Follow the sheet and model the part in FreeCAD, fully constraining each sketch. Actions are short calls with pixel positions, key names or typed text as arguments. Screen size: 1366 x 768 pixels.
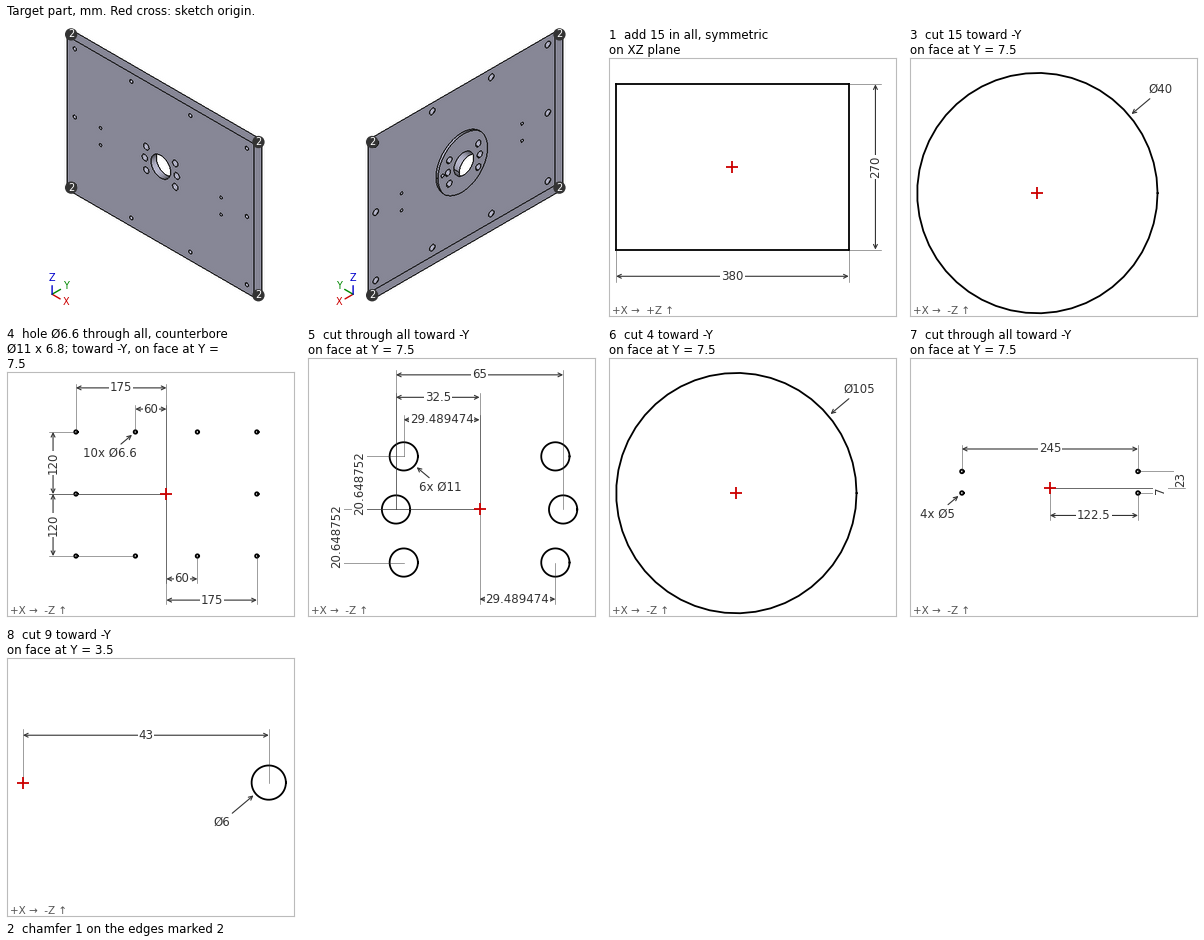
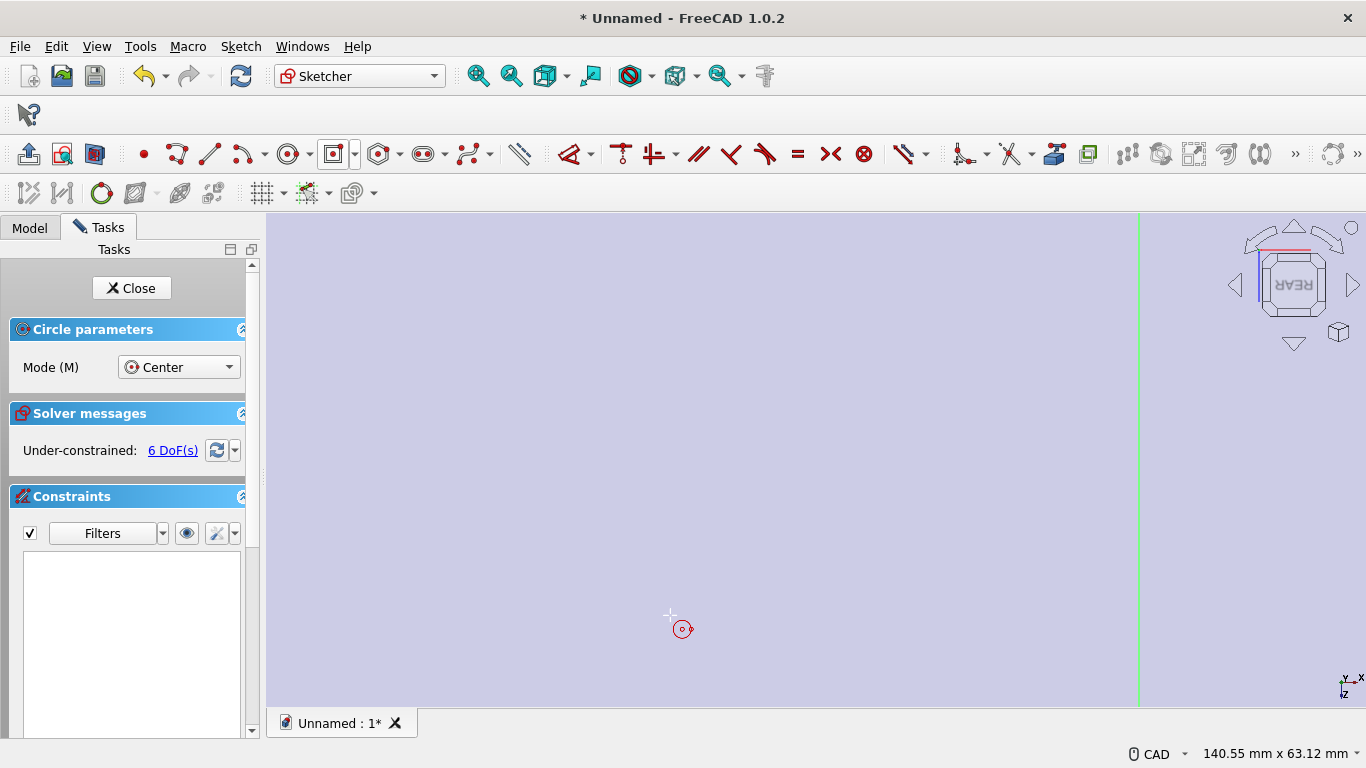
scroll(670, 616, down, 9)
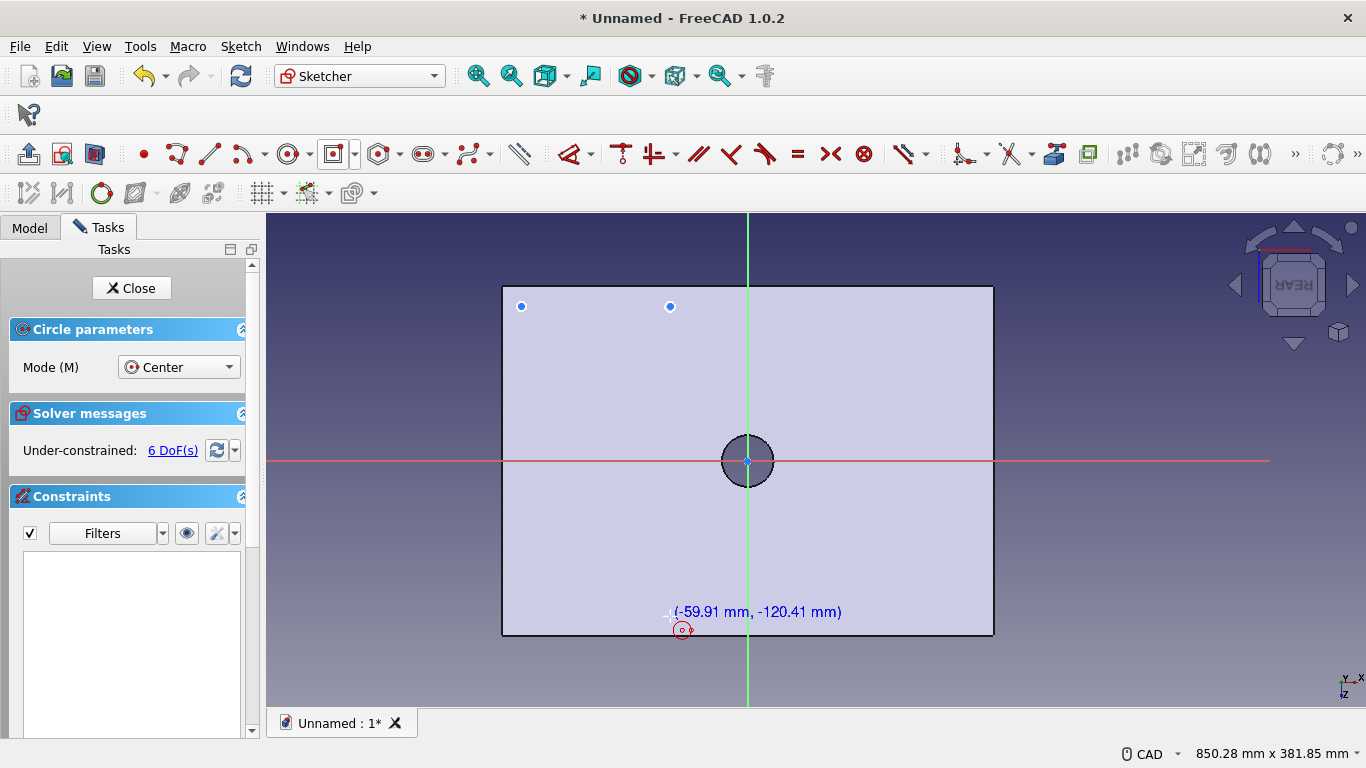
click(670, 616)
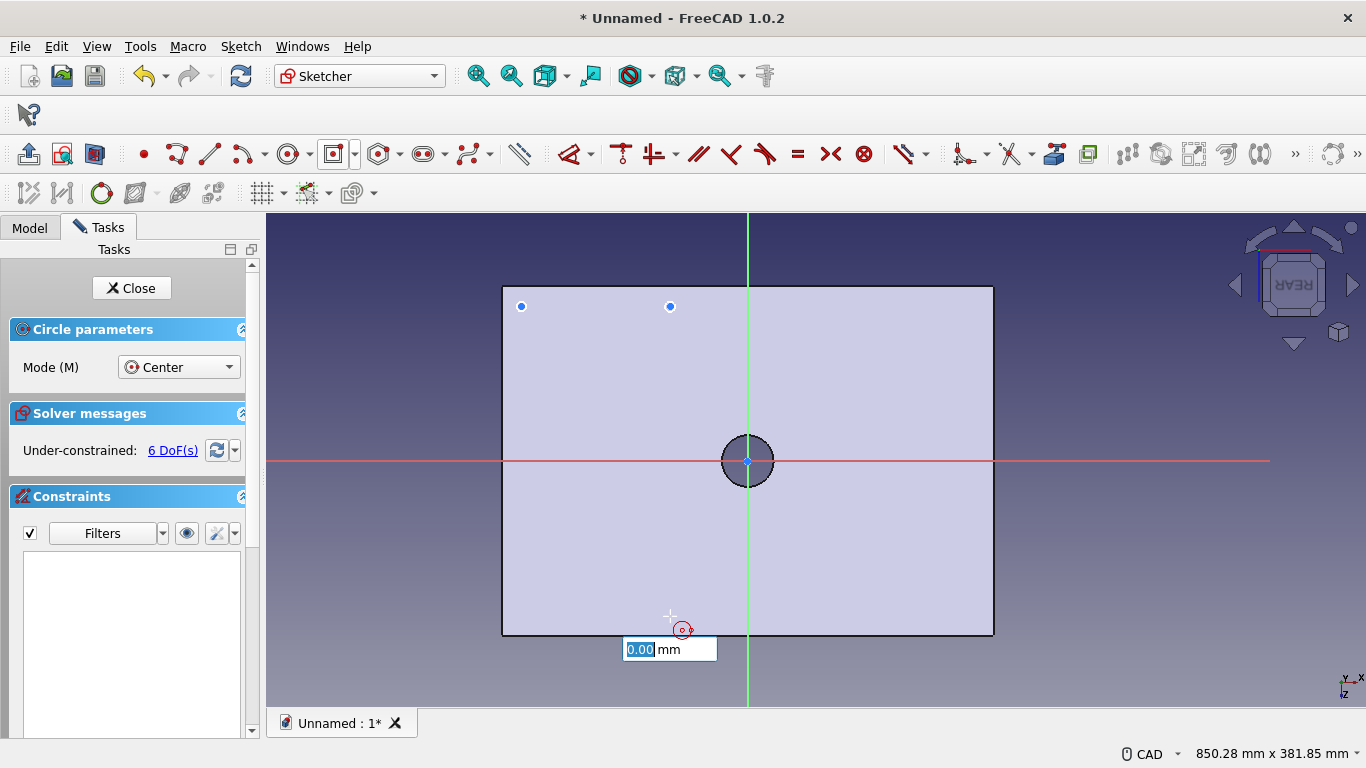
scroll(673, 613, up, 7)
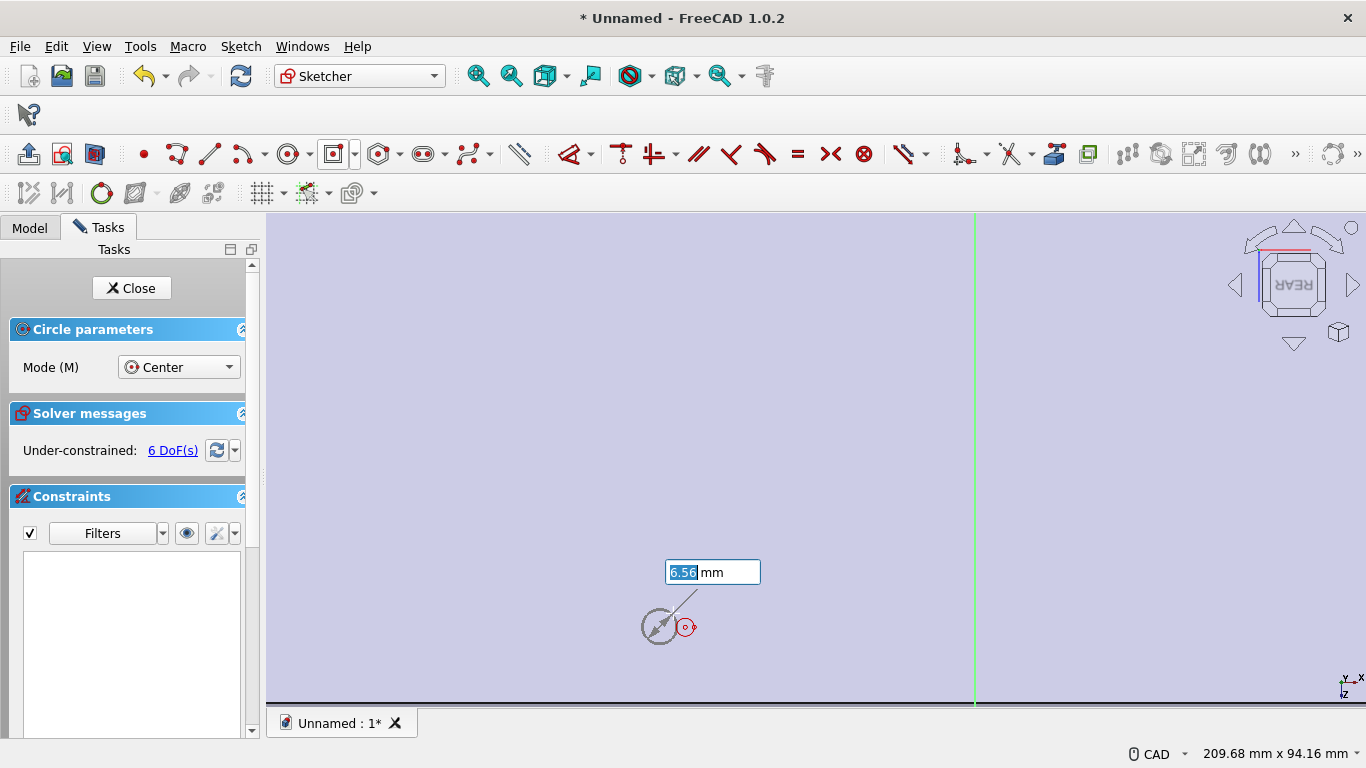
click(673, 612)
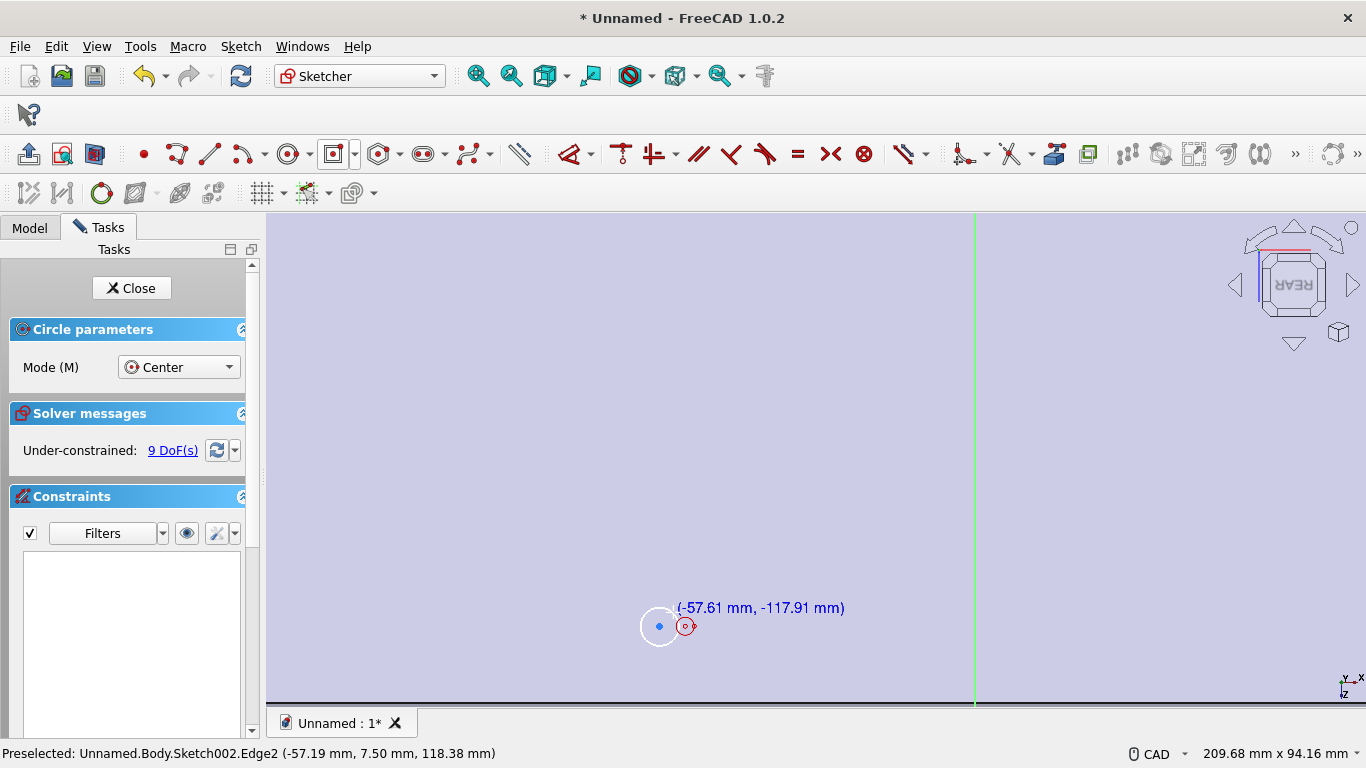
scroll(673, 612, down, 7)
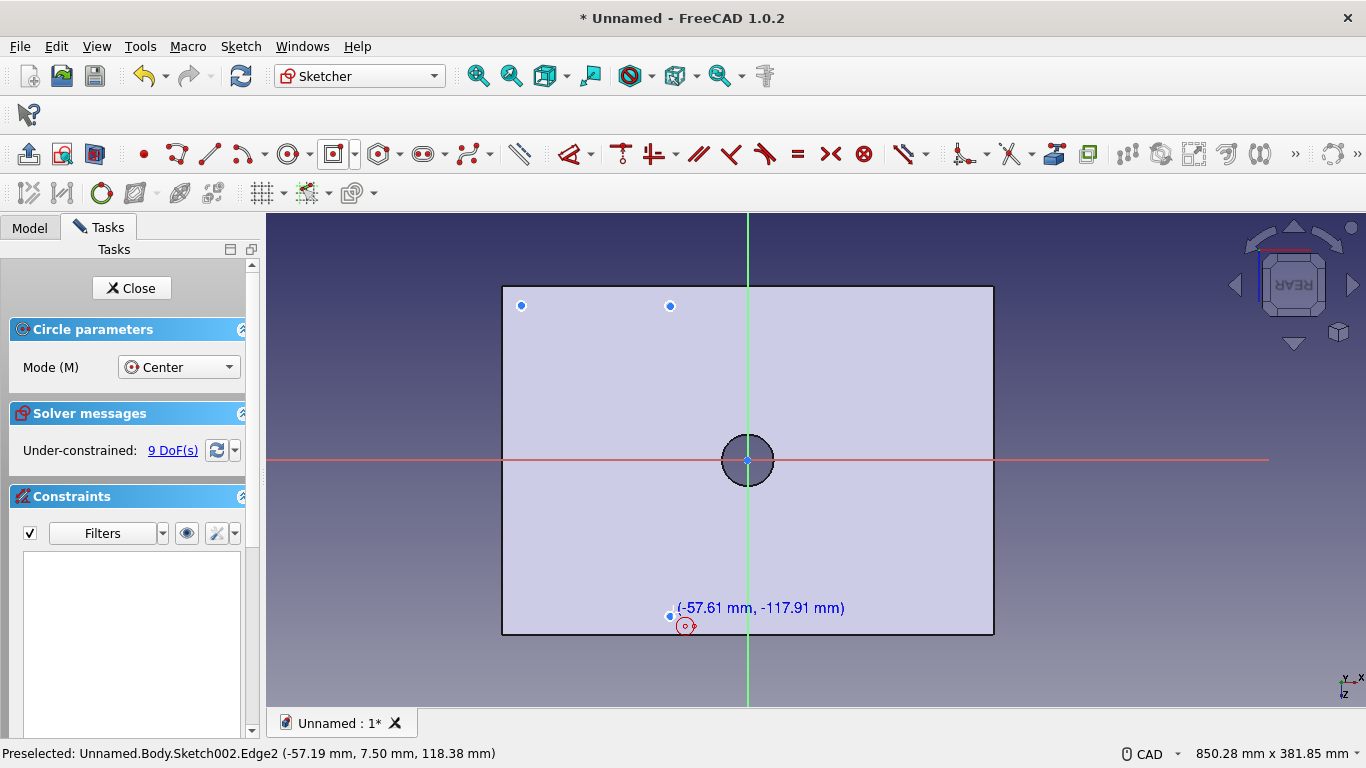
scroll(521, 460, up, 9)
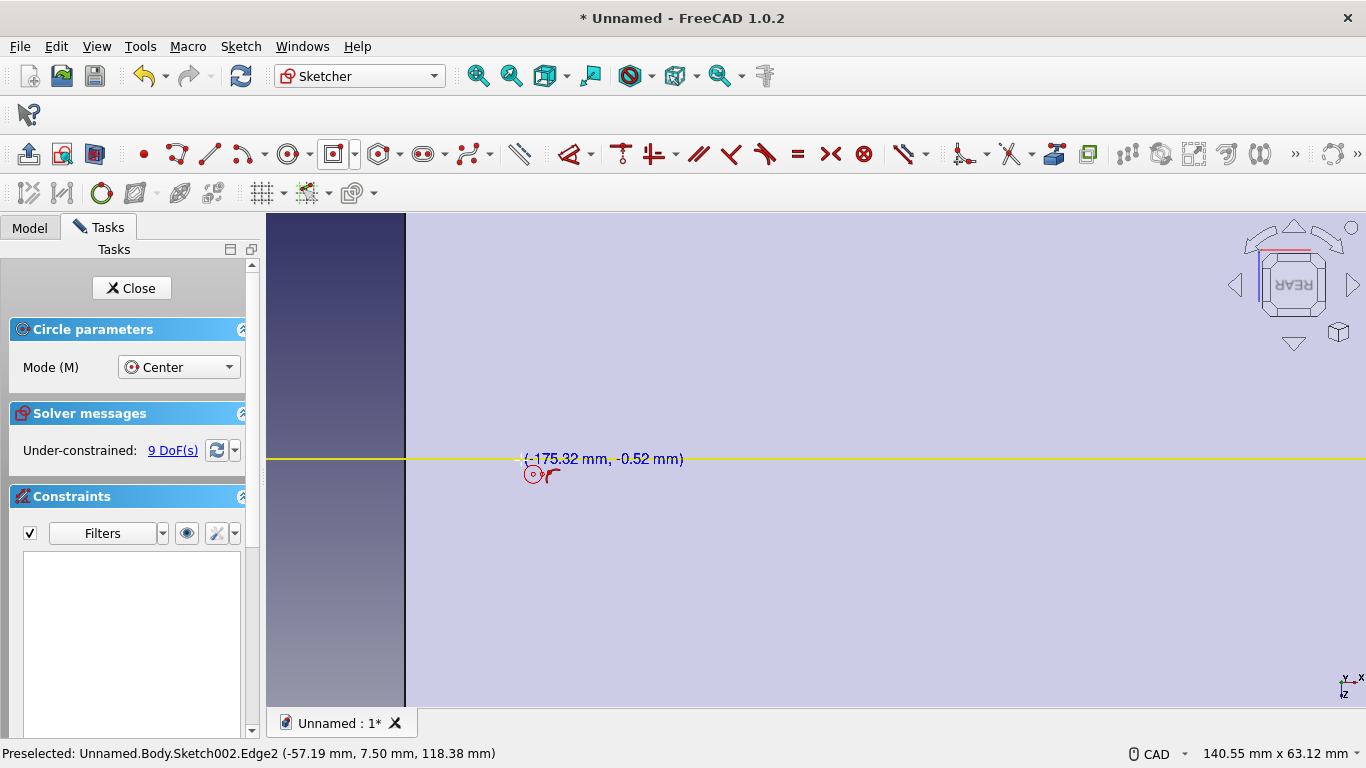
scroll(521, 460, down, 9)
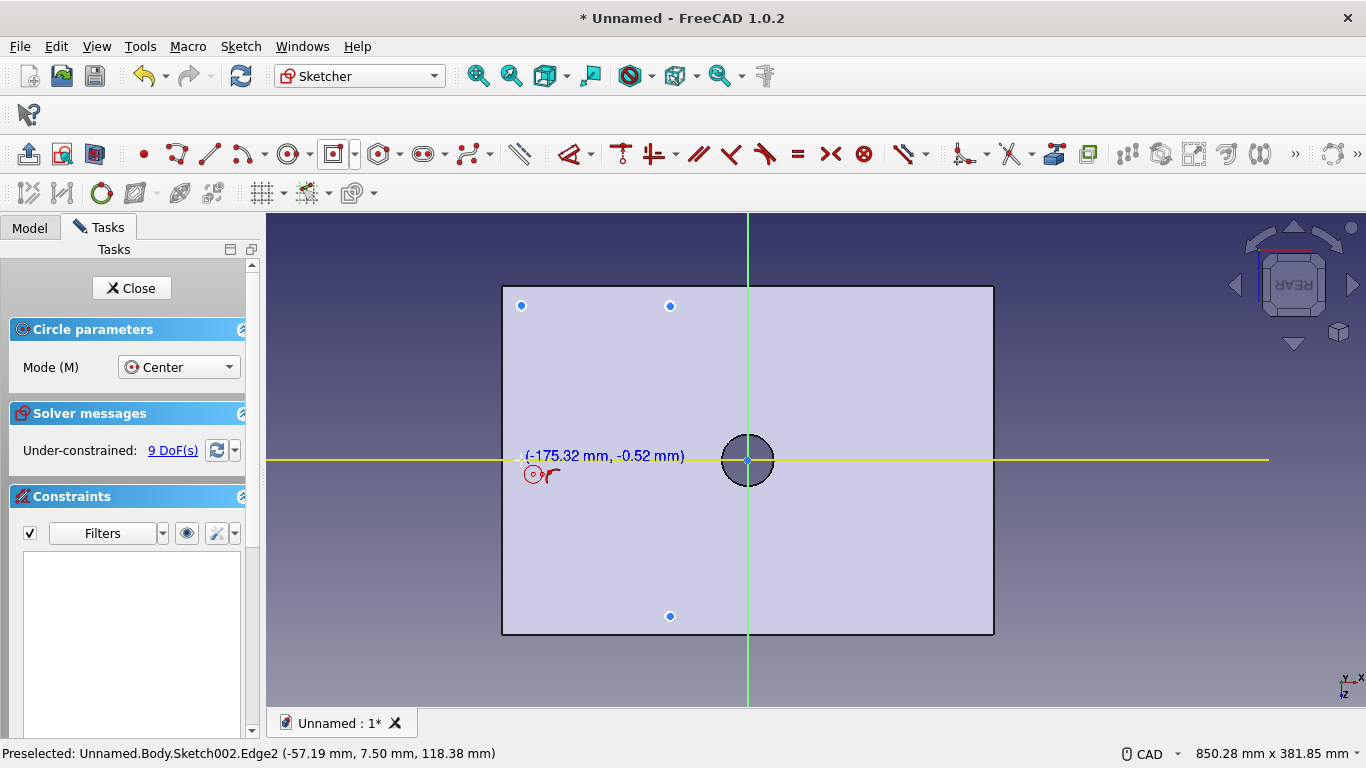
click(521, 460)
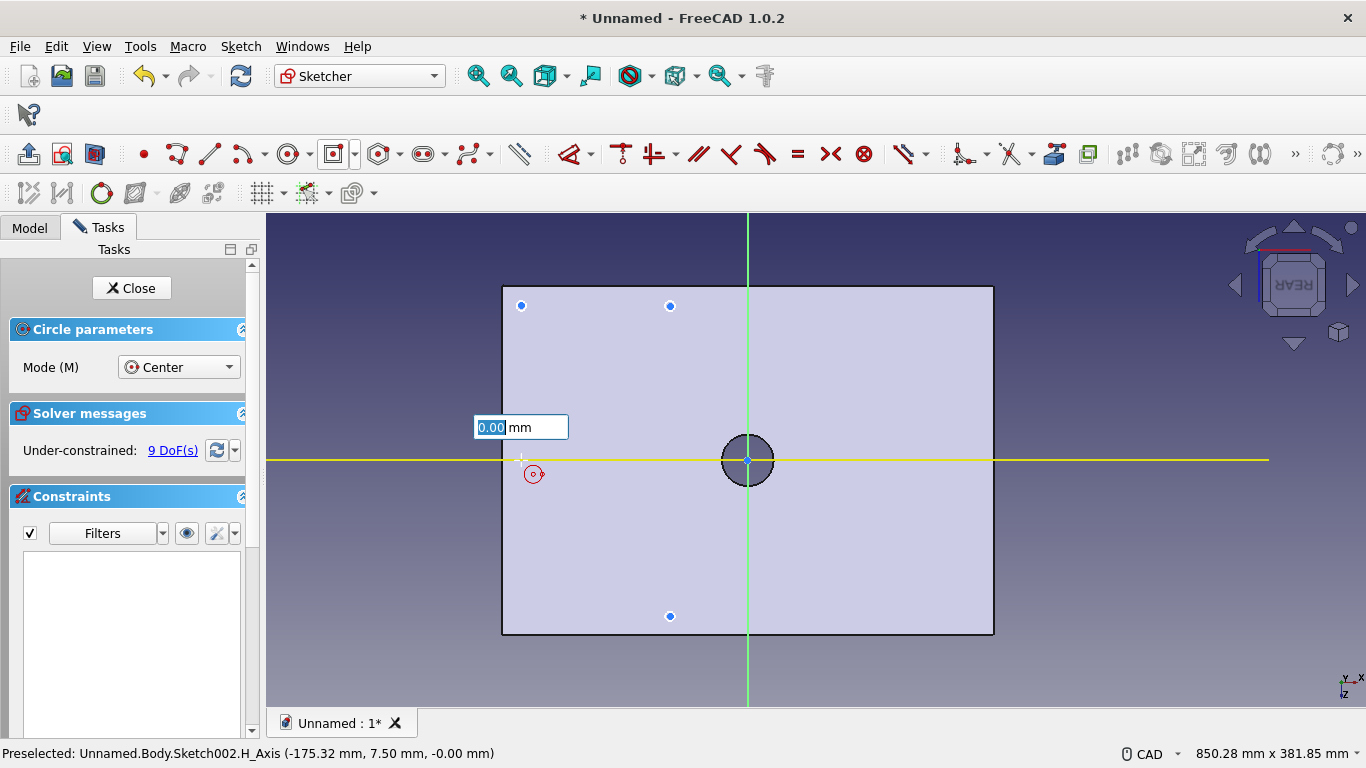
scroll(520, 464, up, 7)